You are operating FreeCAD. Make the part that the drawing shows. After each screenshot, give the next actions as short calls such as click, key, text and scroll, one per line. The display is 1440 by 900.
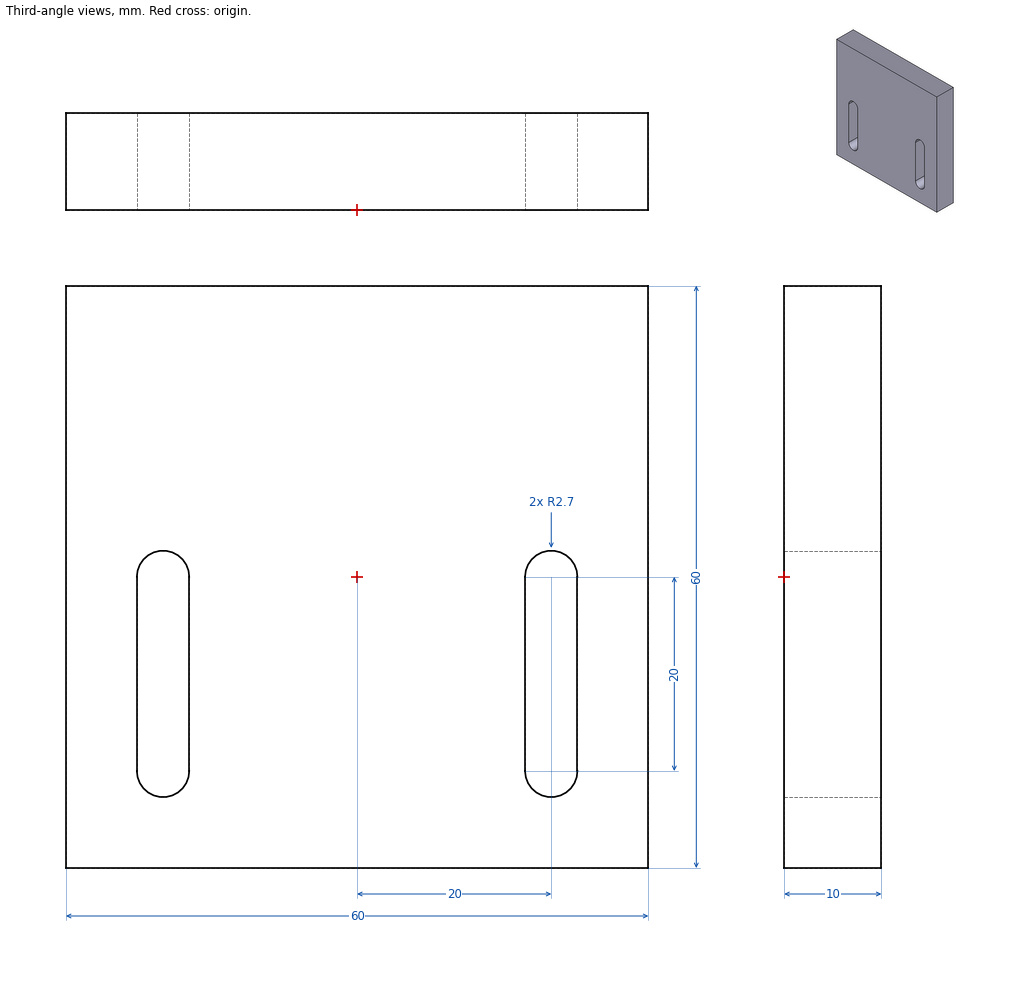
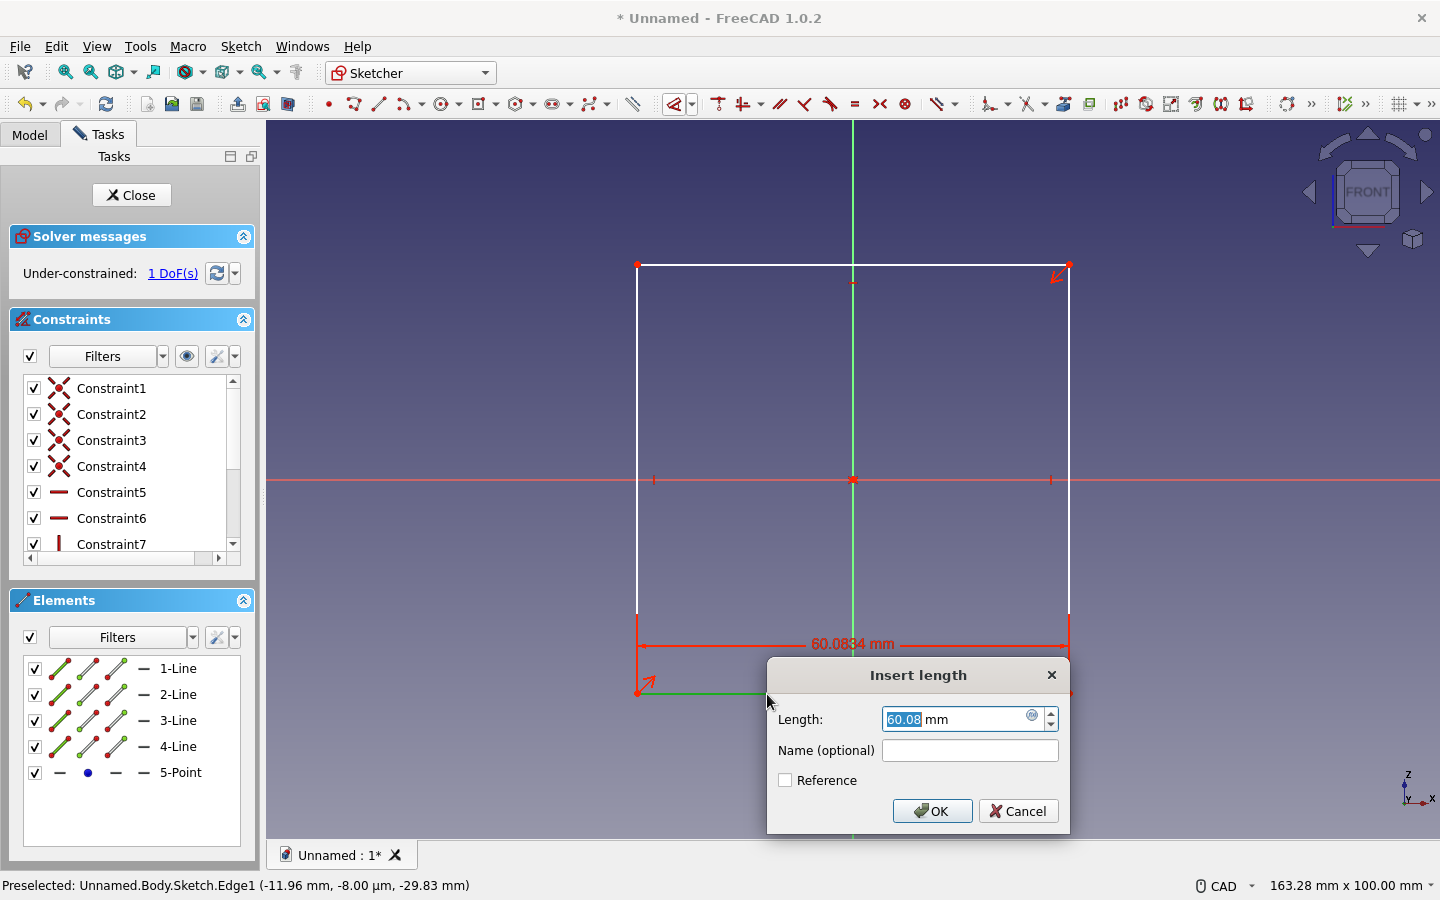
text(60)
key(Return)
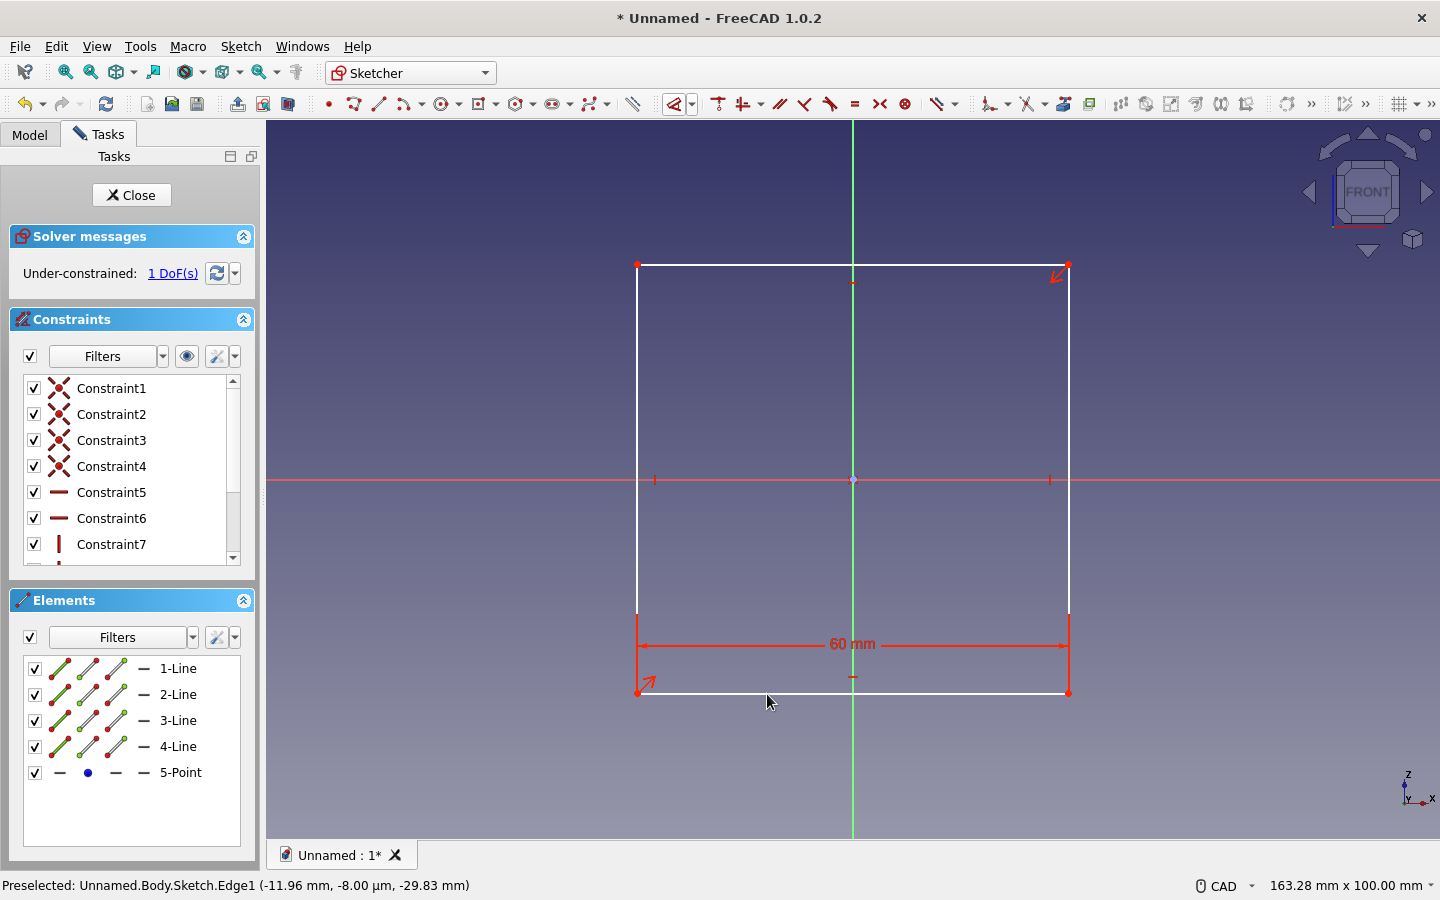
click(1069, 565)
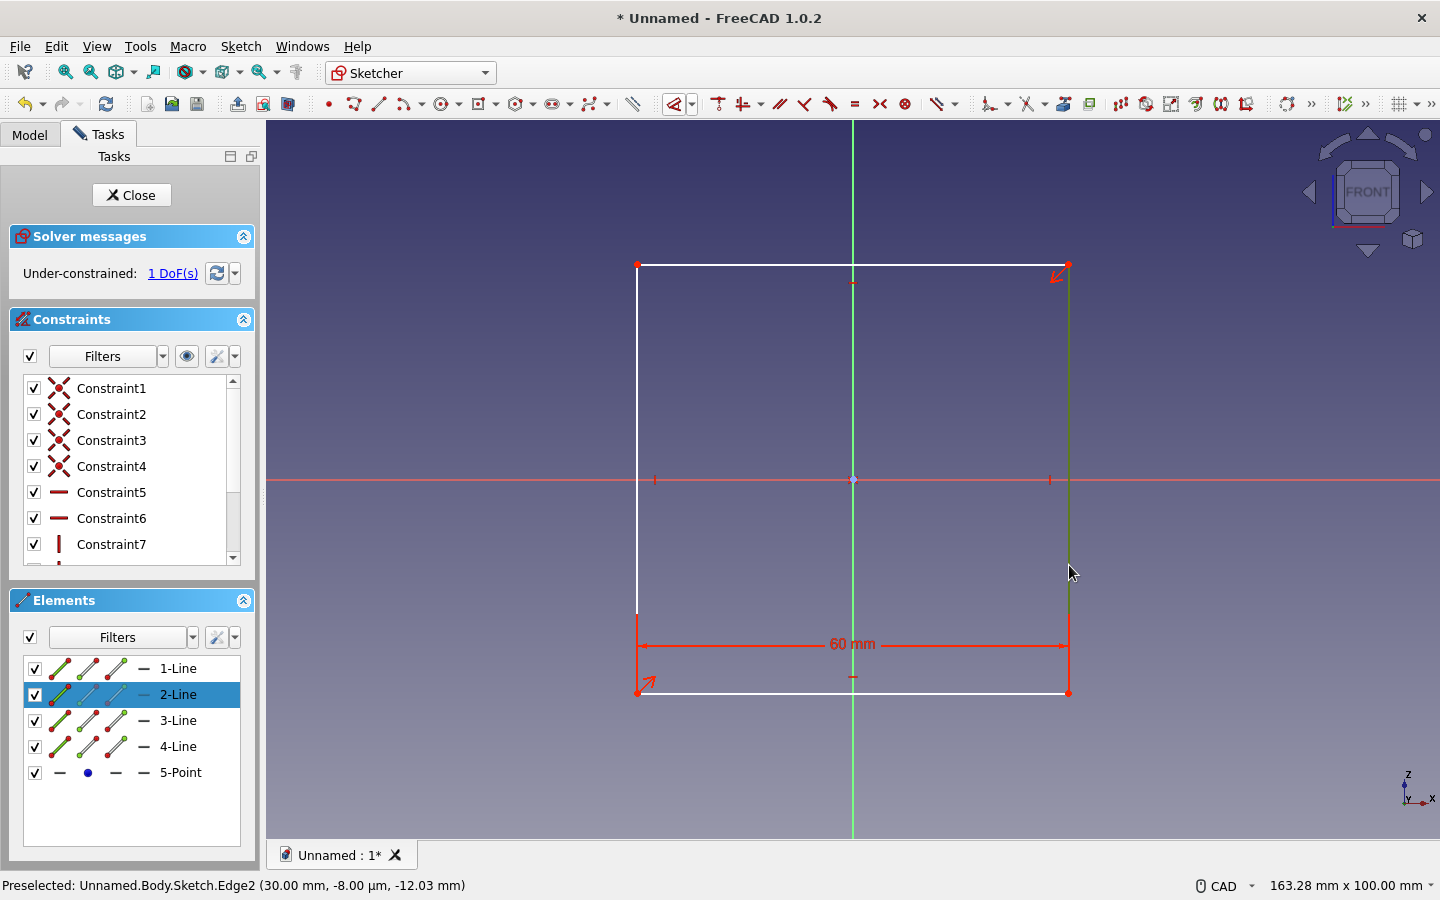
key(i)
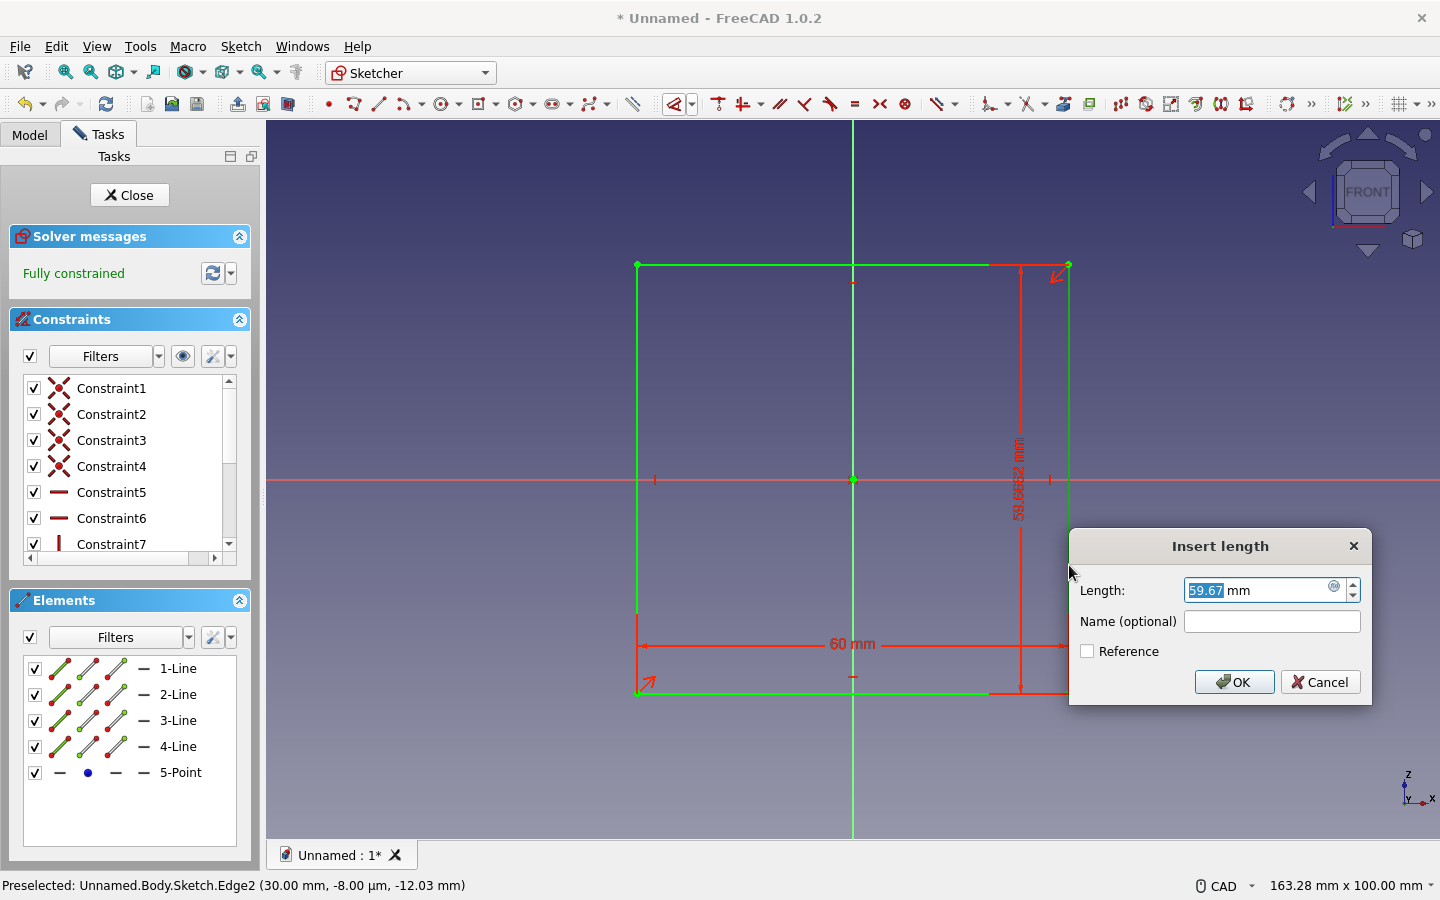
text(60)
key(Return)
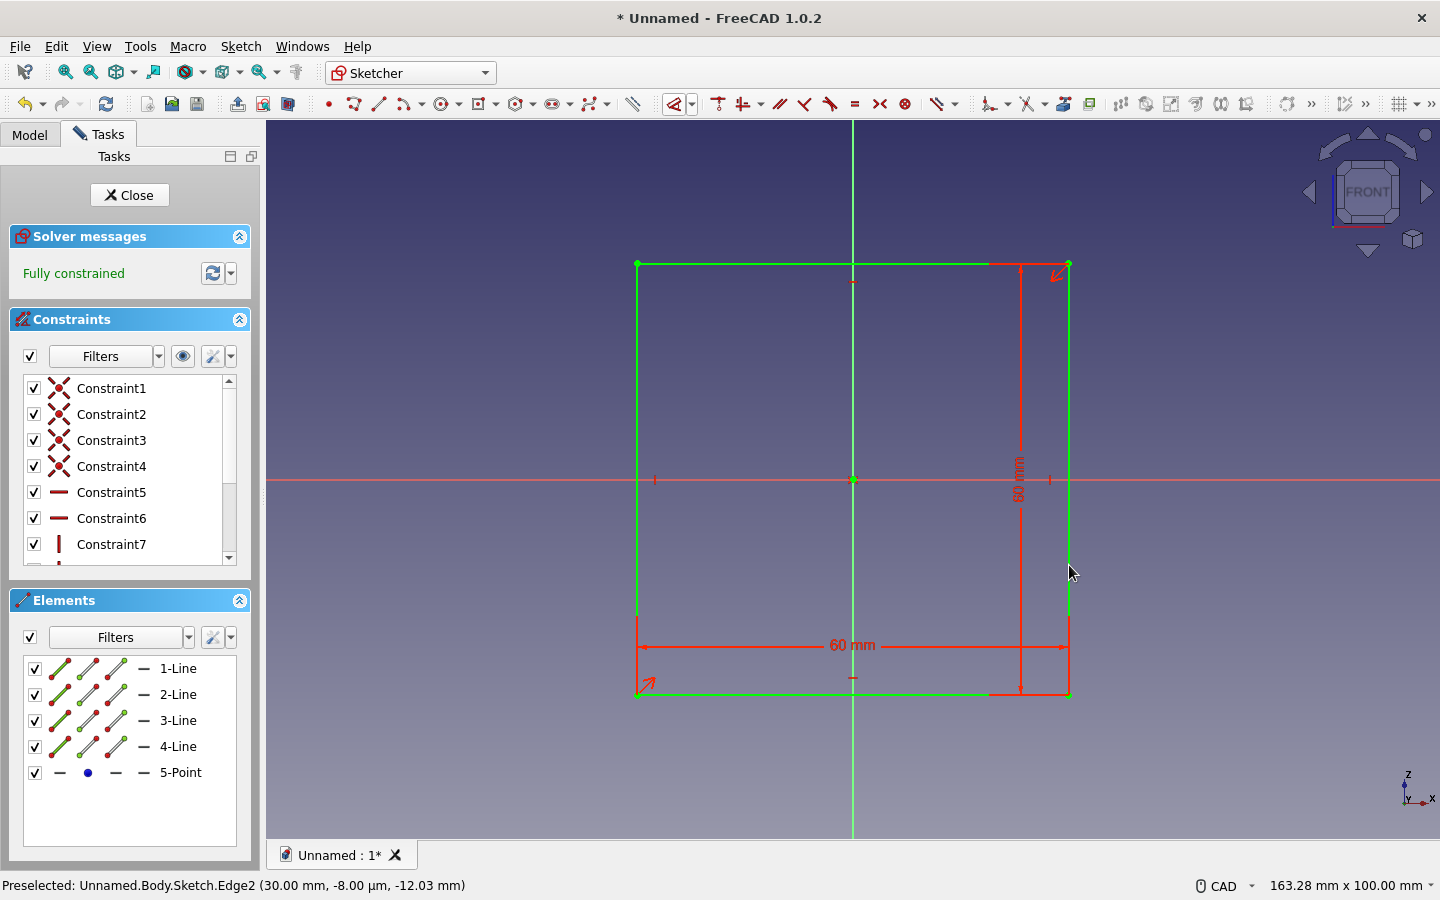
click(130, 195)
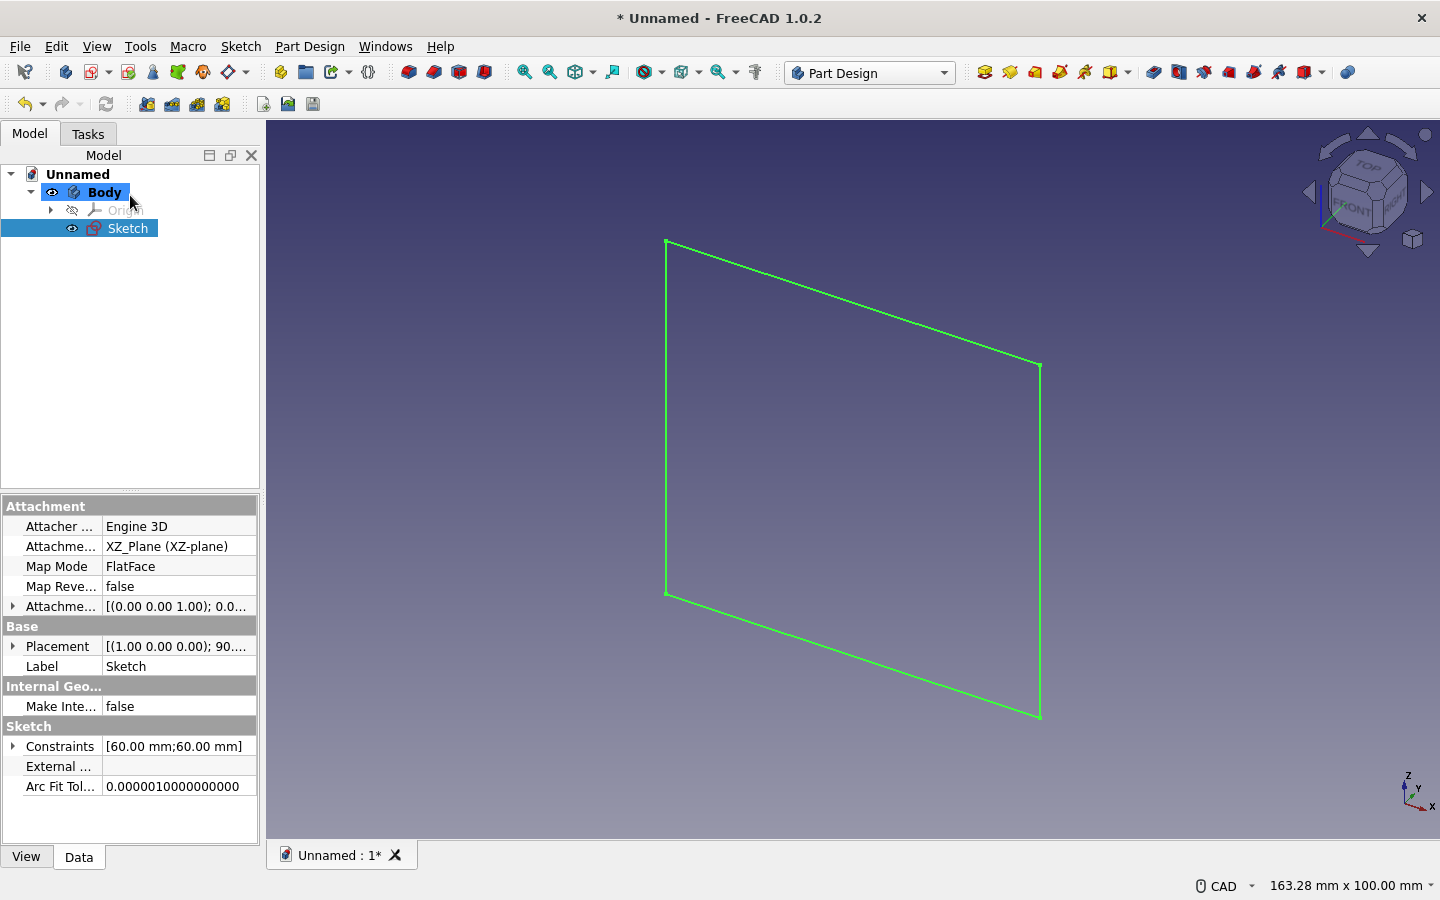
click(985, 72)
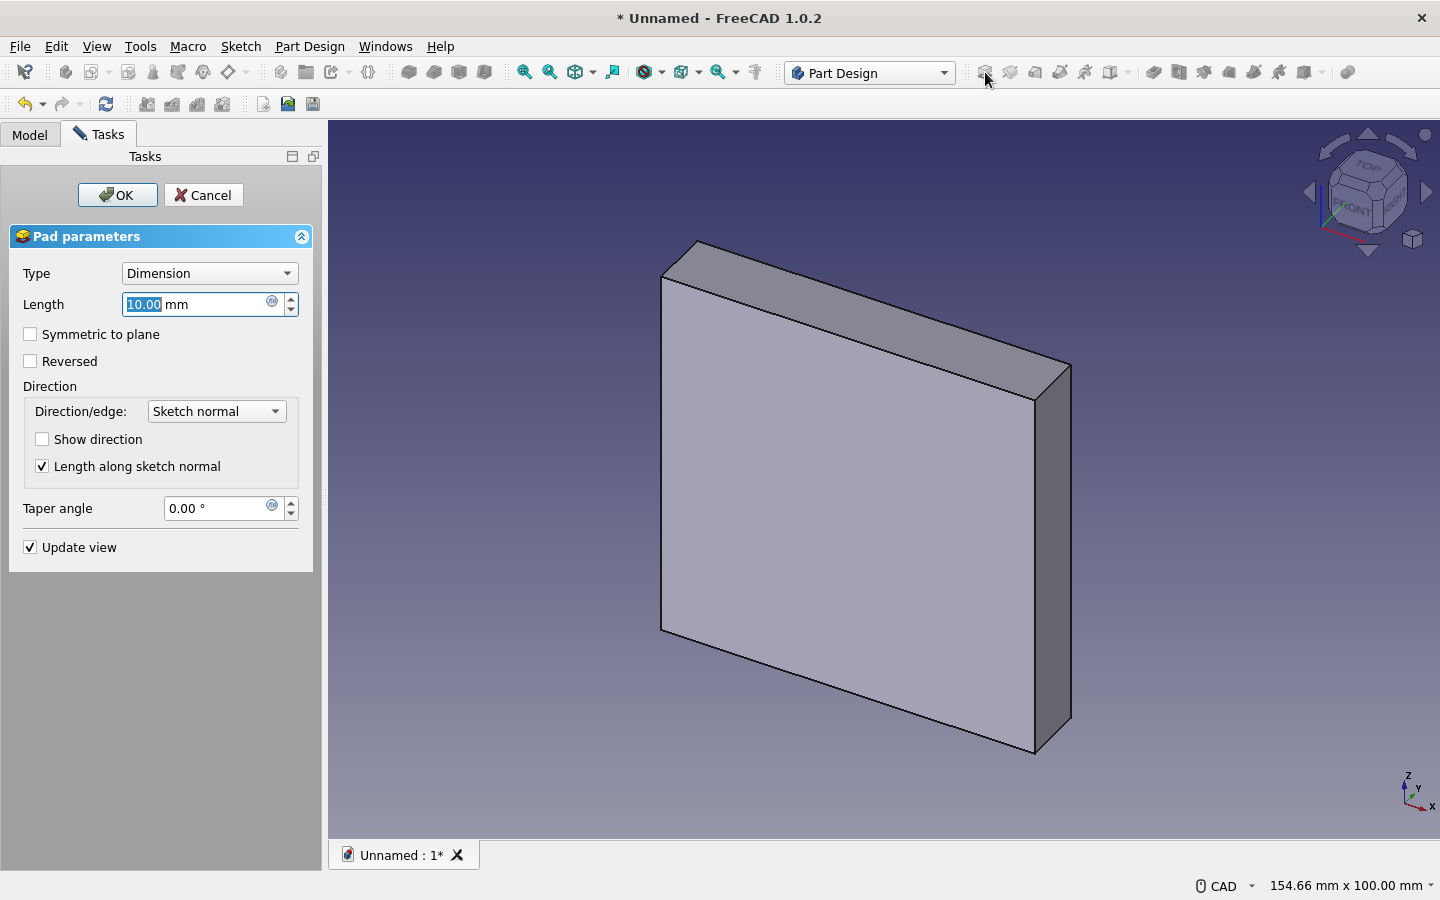
text(10)
key(Tab)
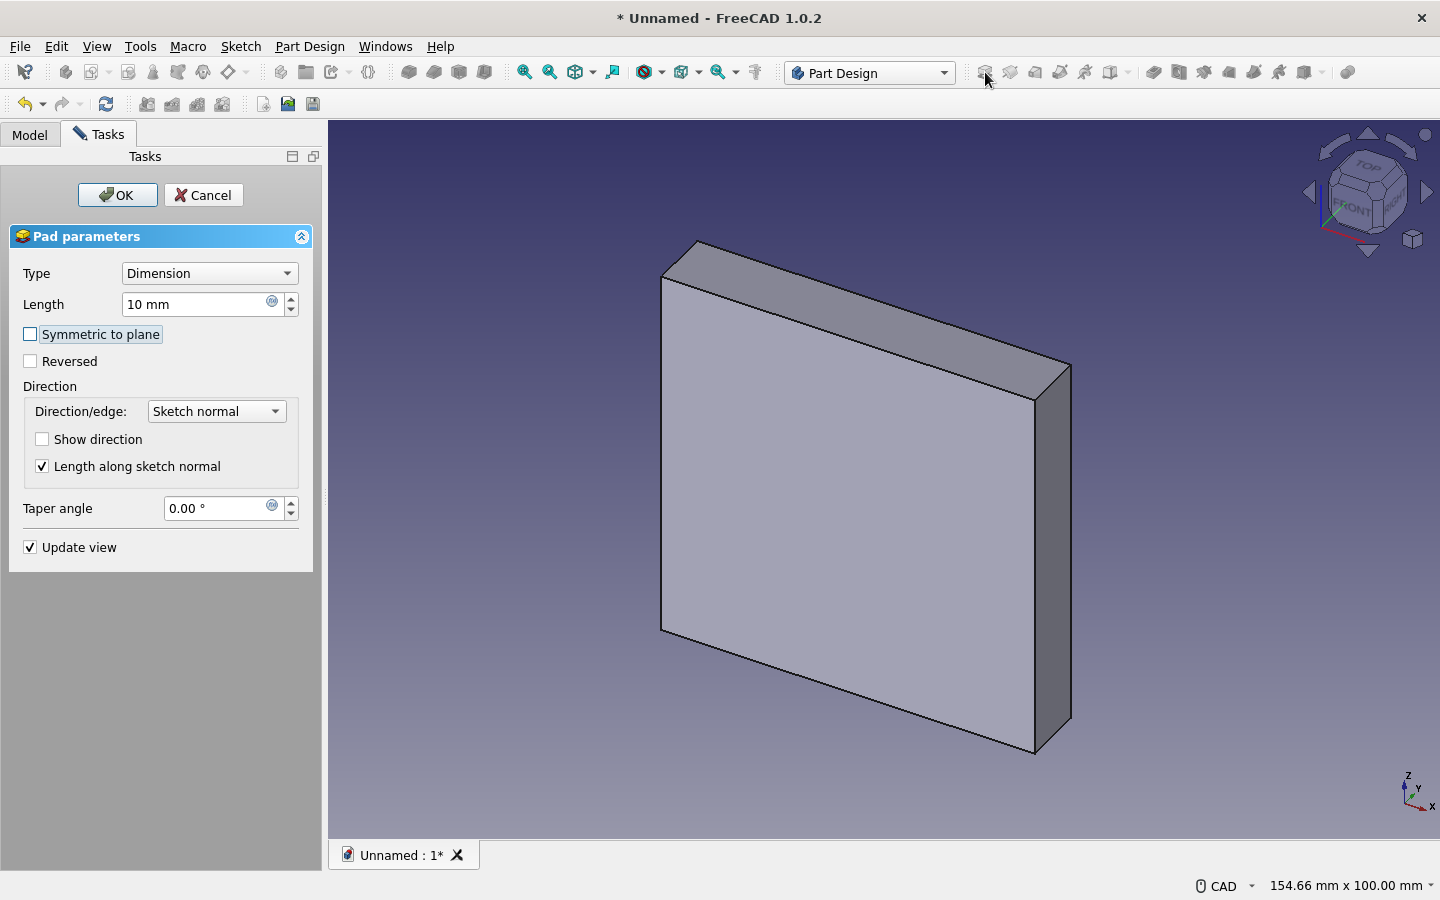
click(31, 361)